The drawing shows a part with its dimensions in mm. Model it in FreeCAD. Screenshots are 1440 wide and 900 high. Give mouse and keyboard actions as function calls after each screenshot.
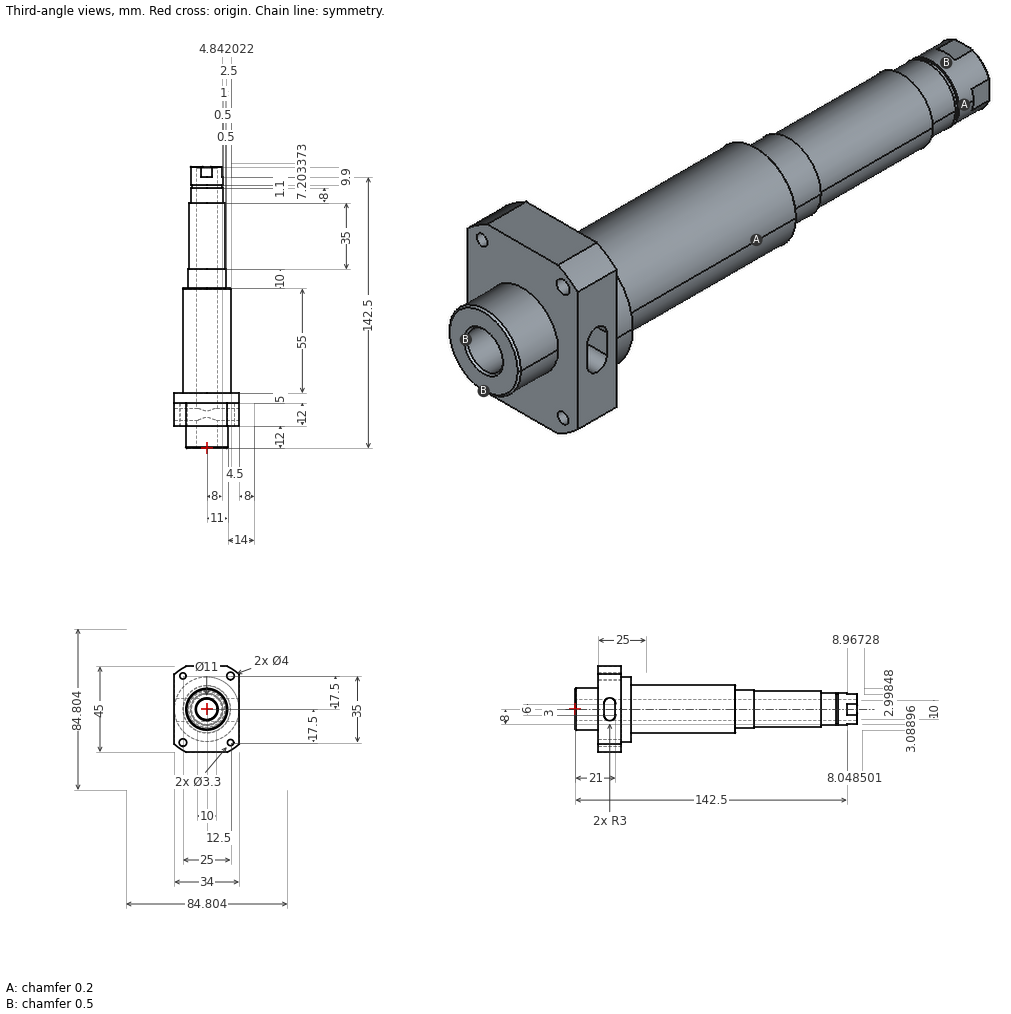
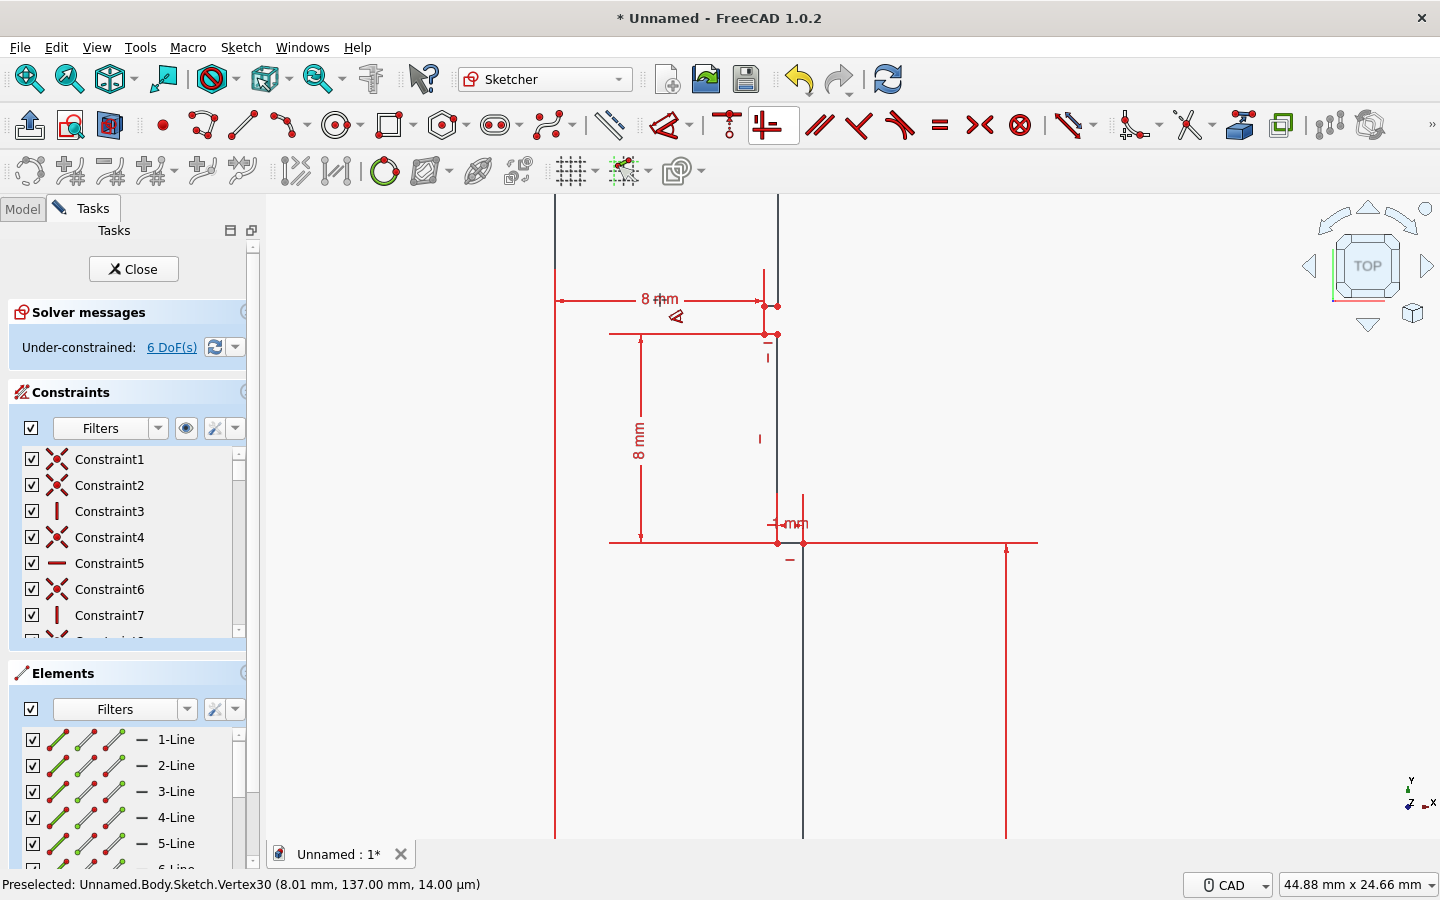
scroll(772, 334, down, 11)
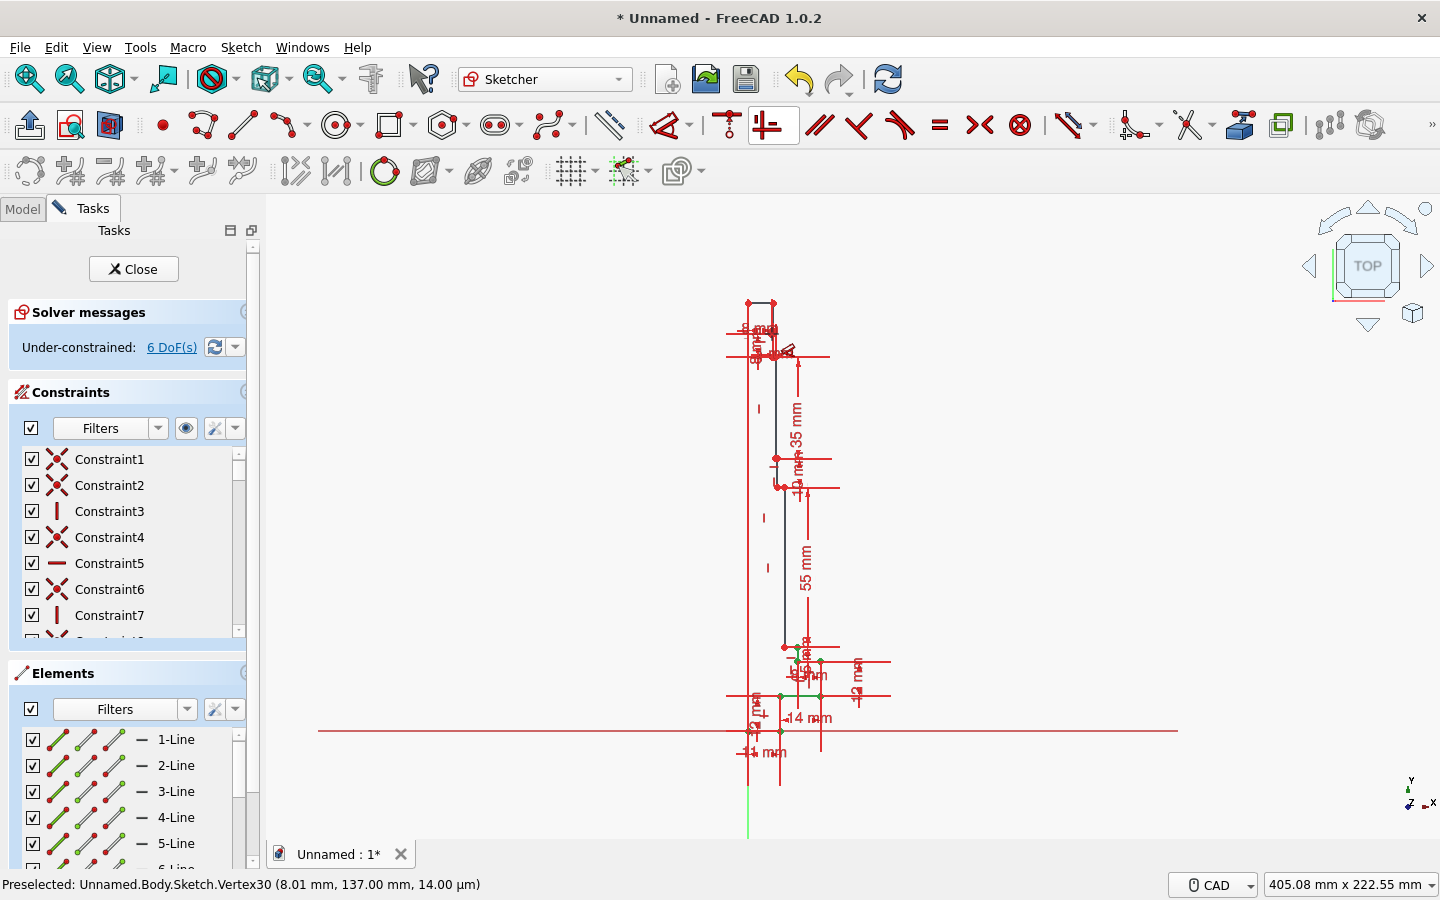
scroll(794, 647, up, 7)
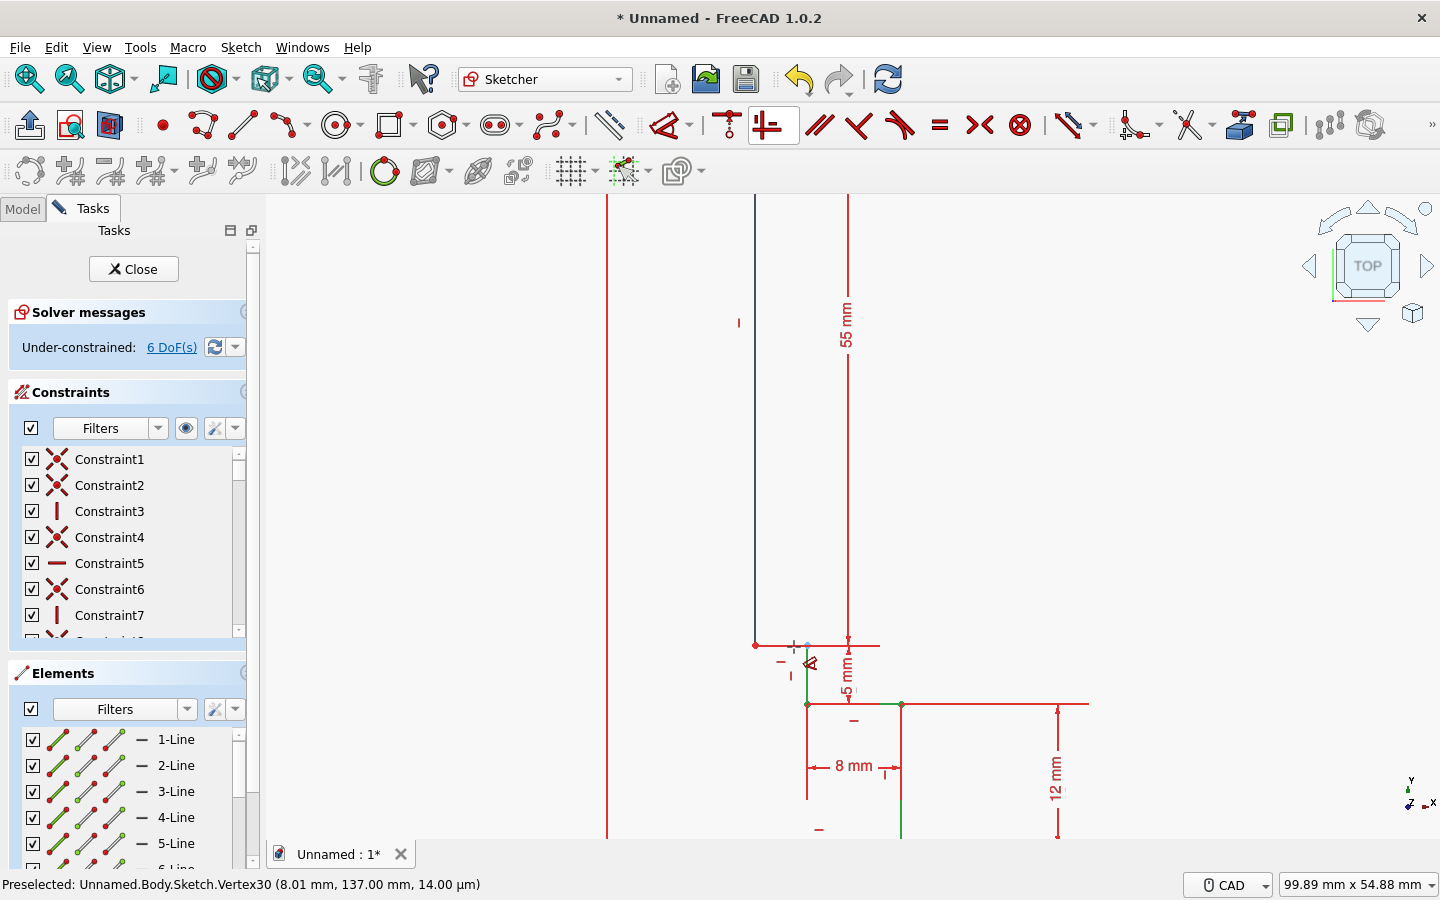
click(792, 646)
click(769, 680)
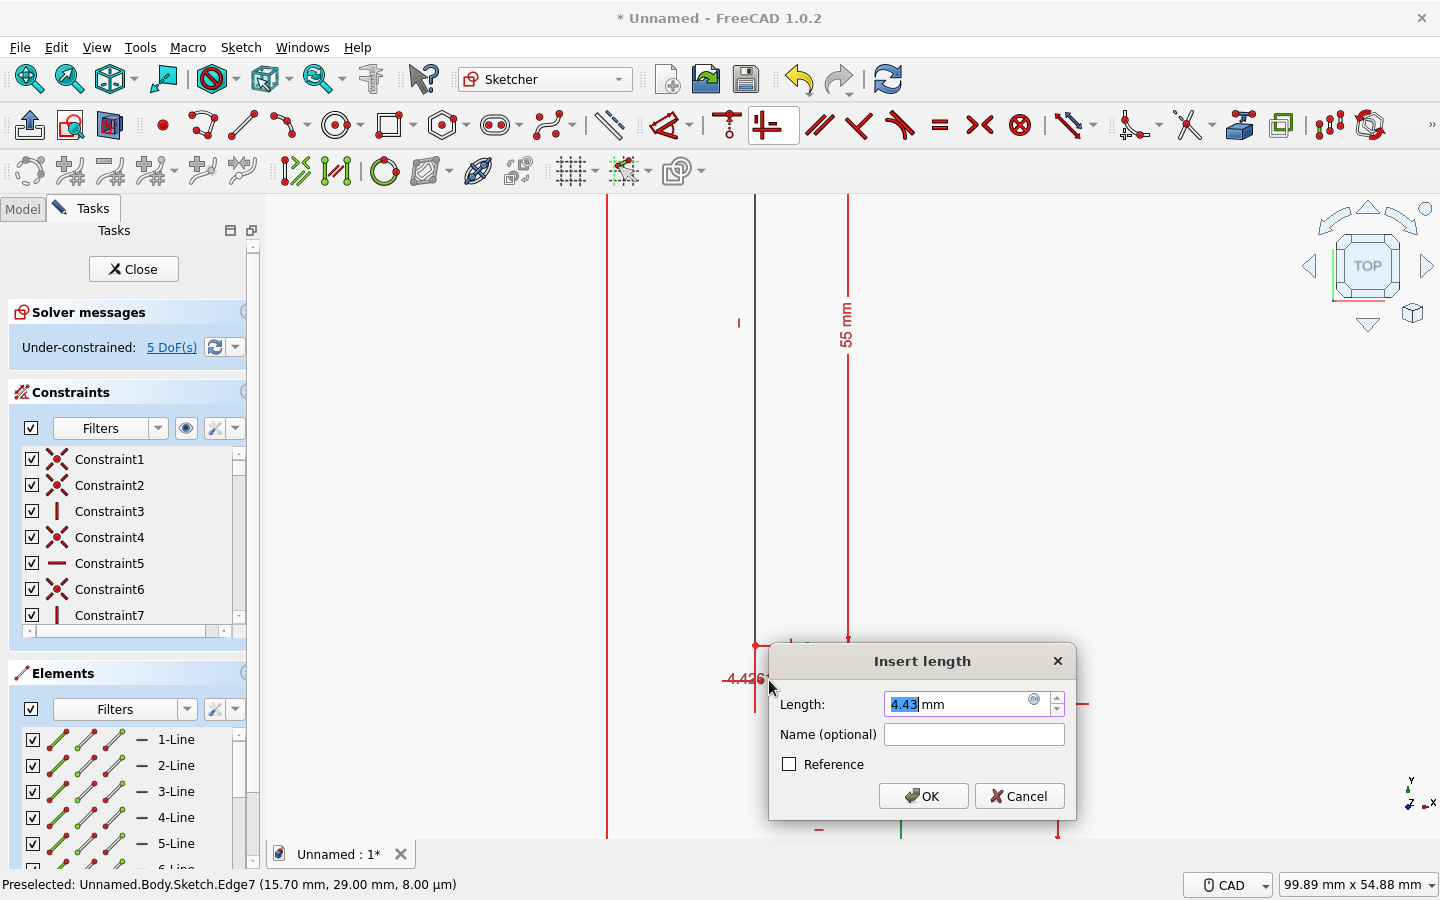
text(4.5)
key(Return)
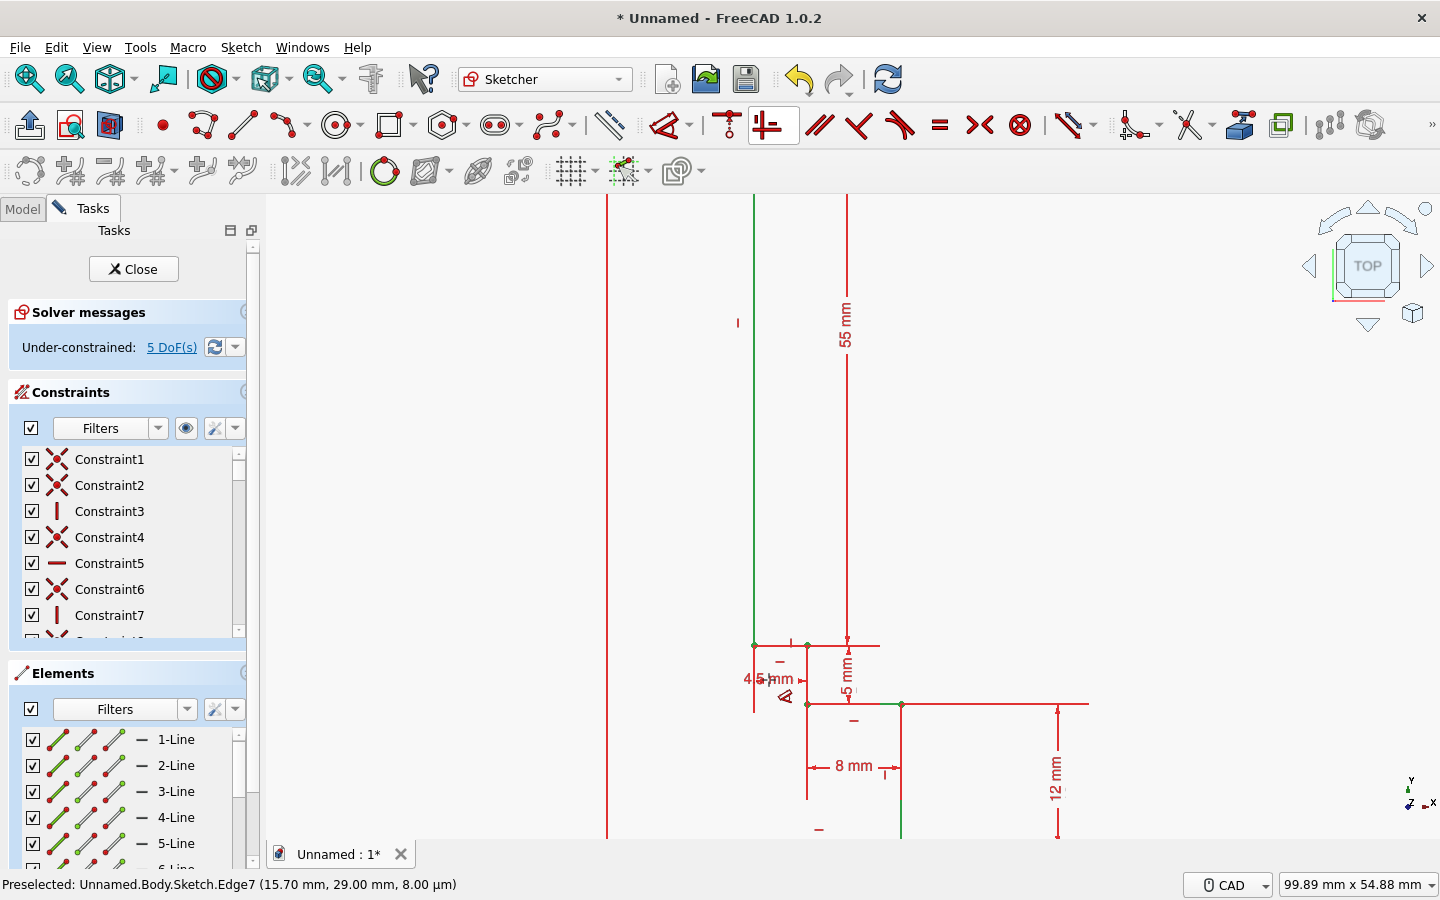
scroll(794, 647, down, 7)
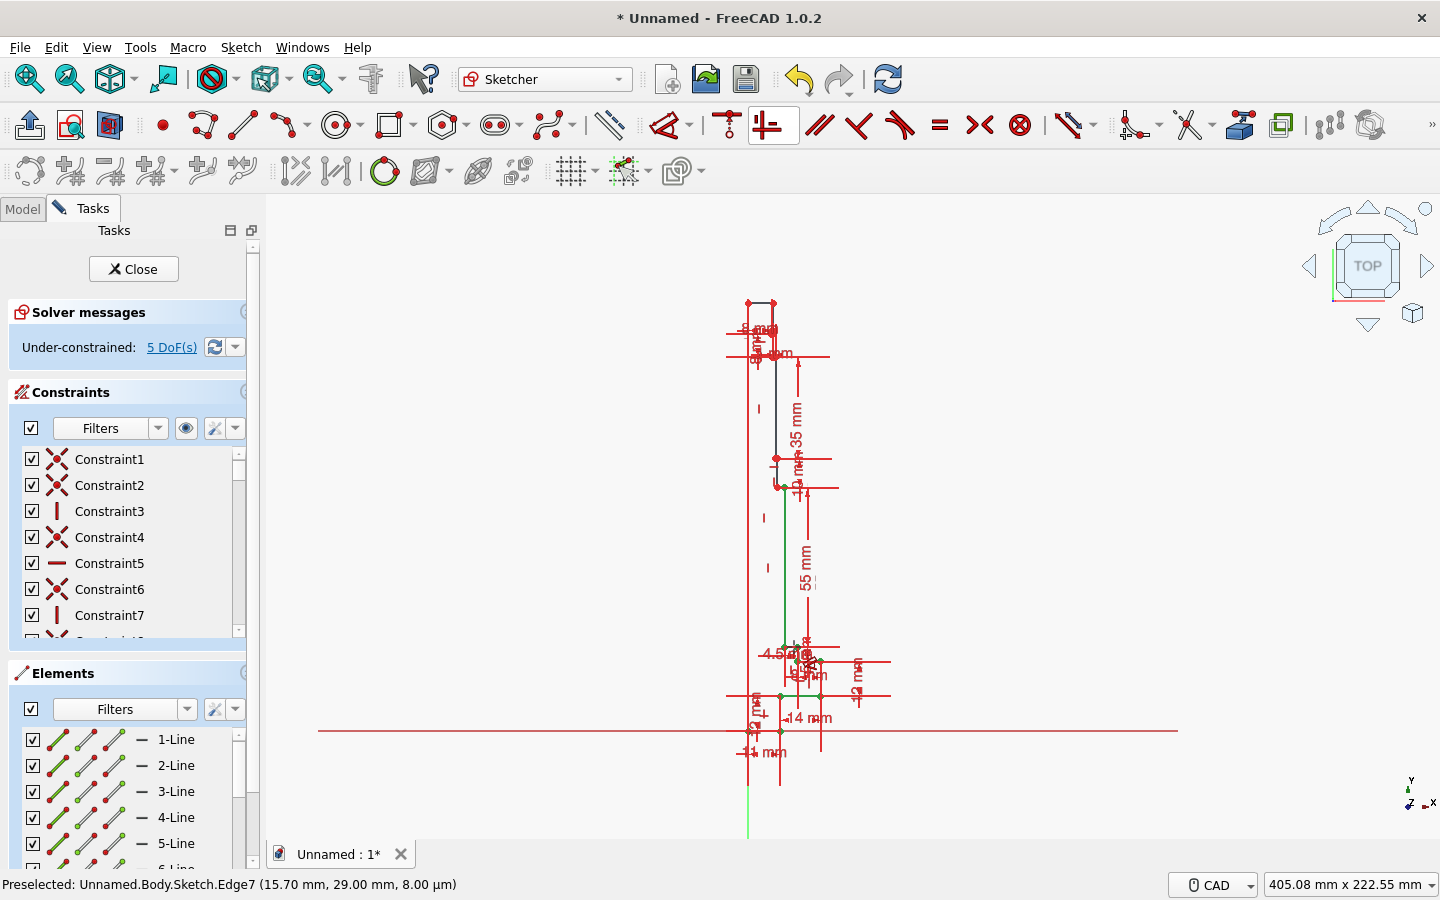
scroll(782, 488, up, 10)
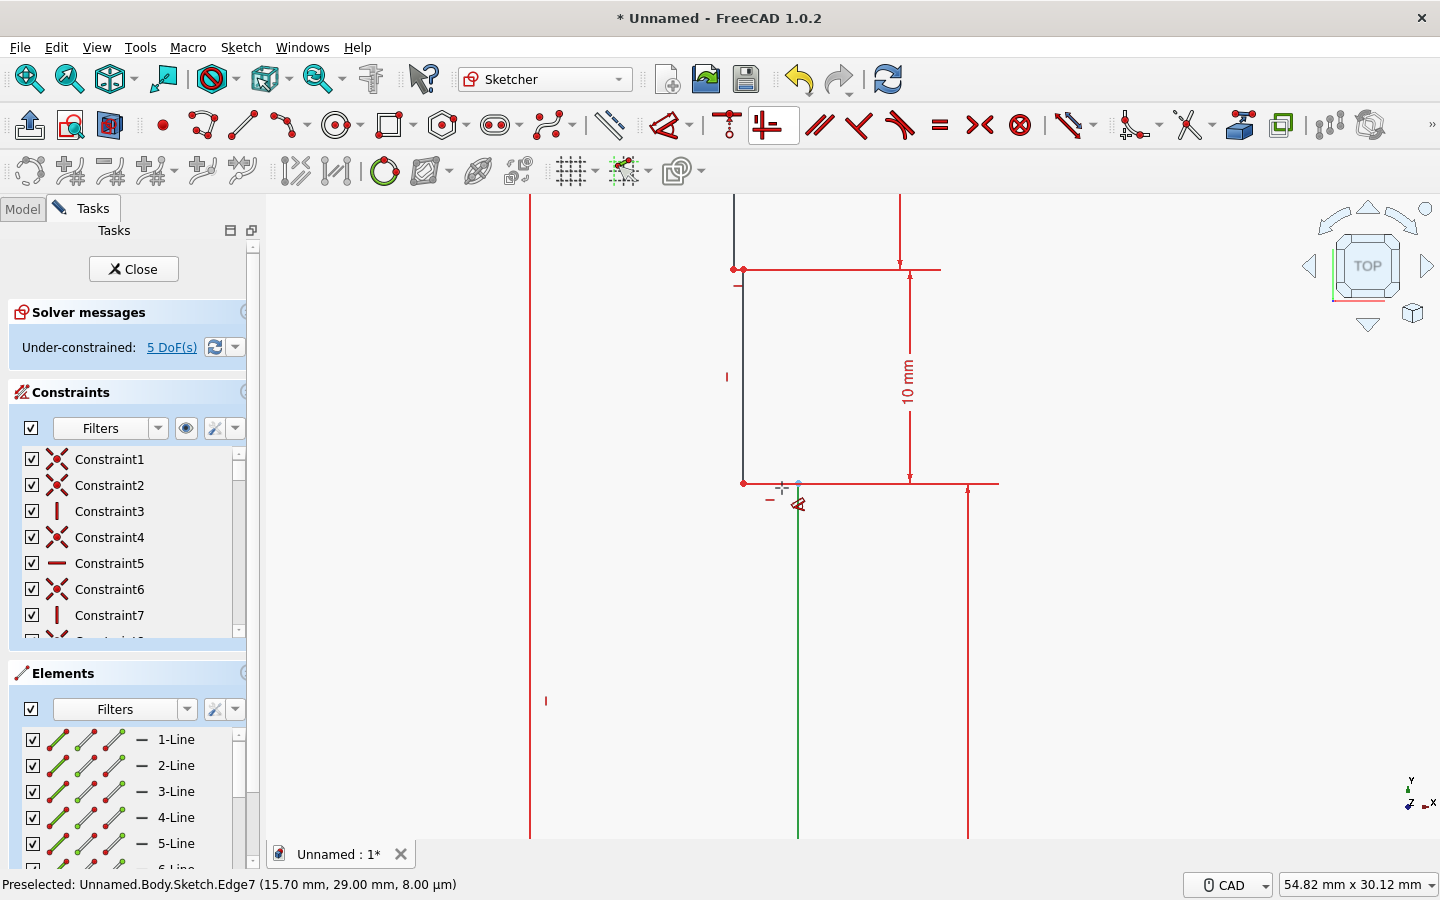
click(782, 484)
click(771, 450)